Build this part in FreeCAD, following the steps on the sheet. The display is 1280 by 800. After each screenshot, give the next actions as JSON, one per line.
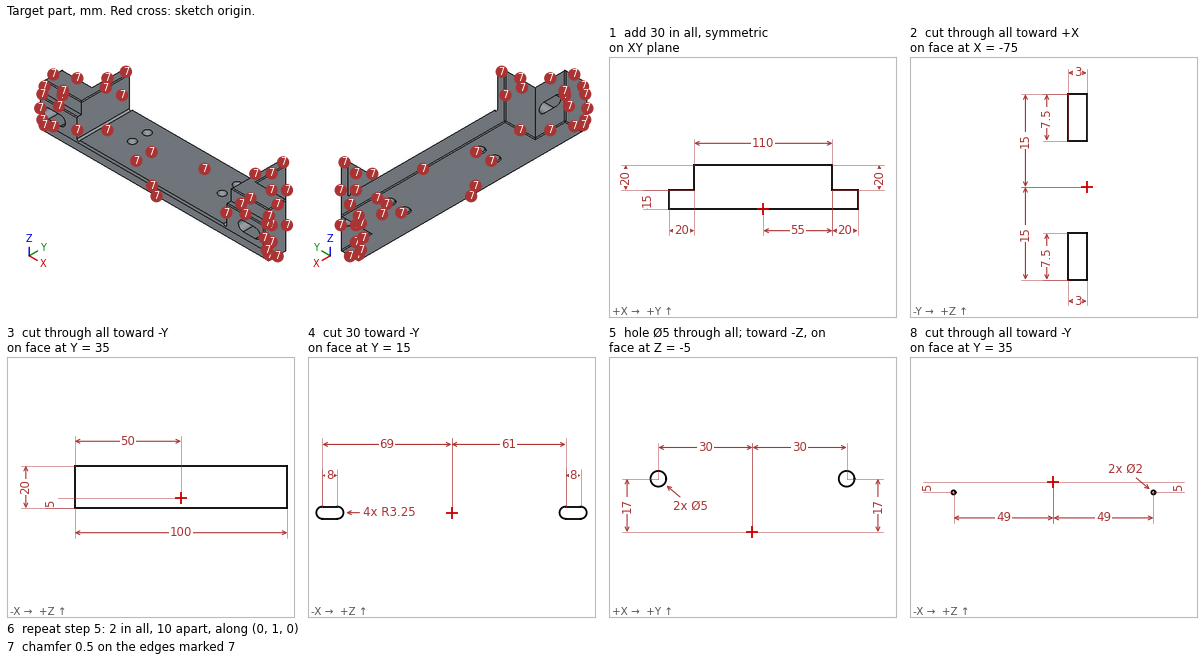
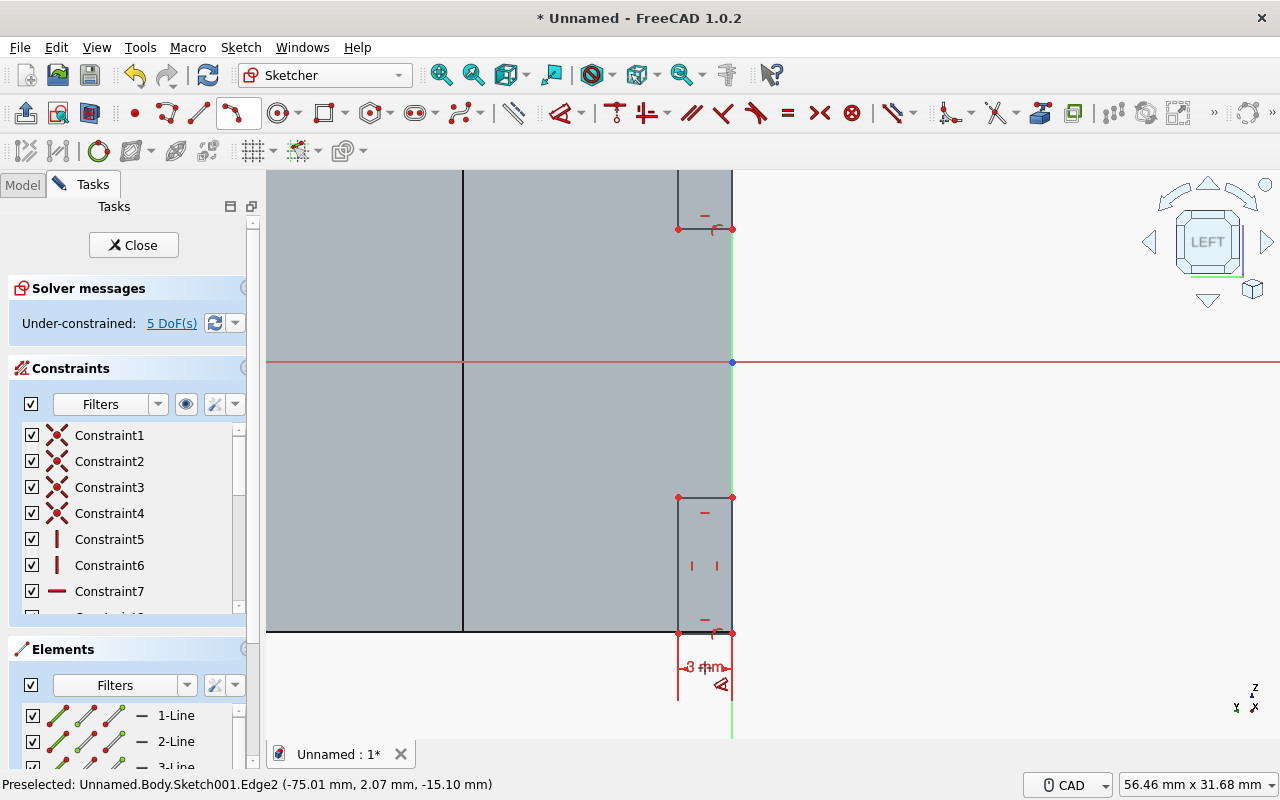
{"action": "left_click", "coordinate": [695, 229]}
{"action": "left_click", "coordinate": [705, 263]}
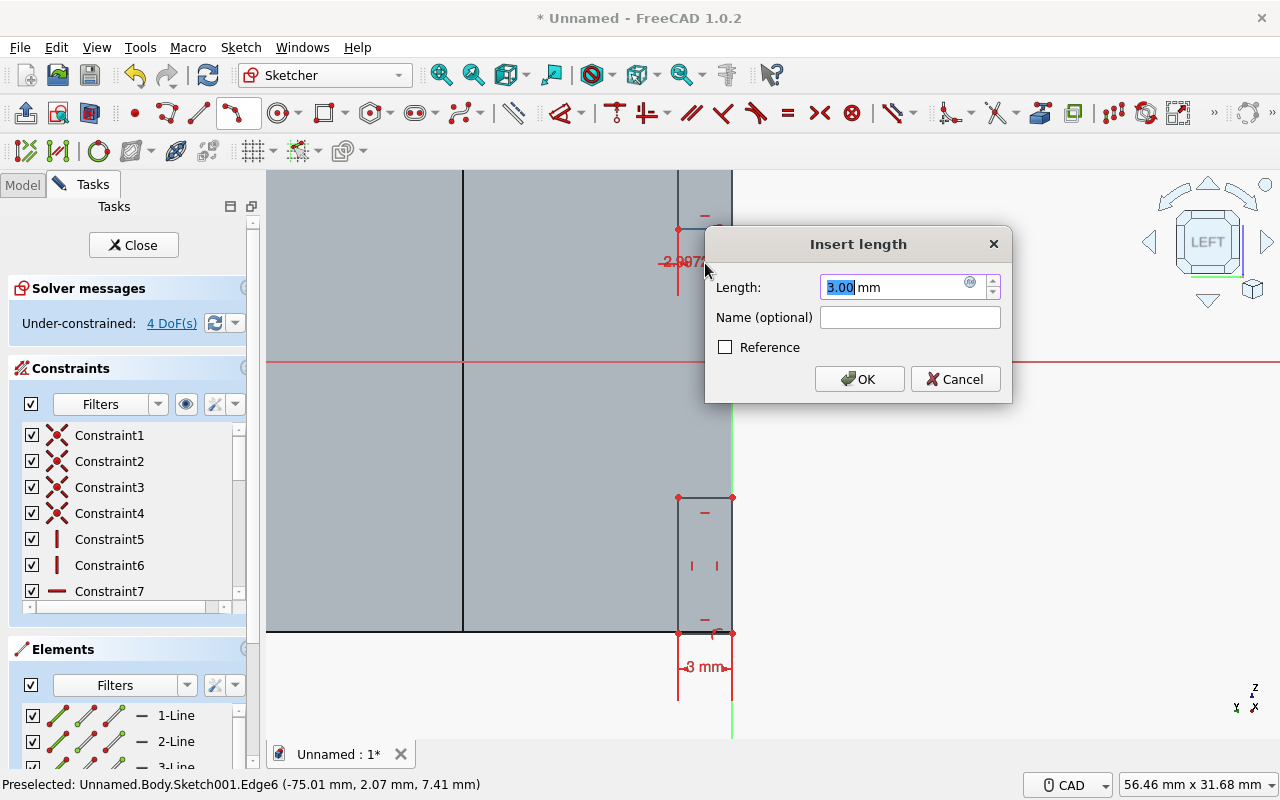
{"action": "type", "text": "3"}
{"action": "key", "text": "Return"}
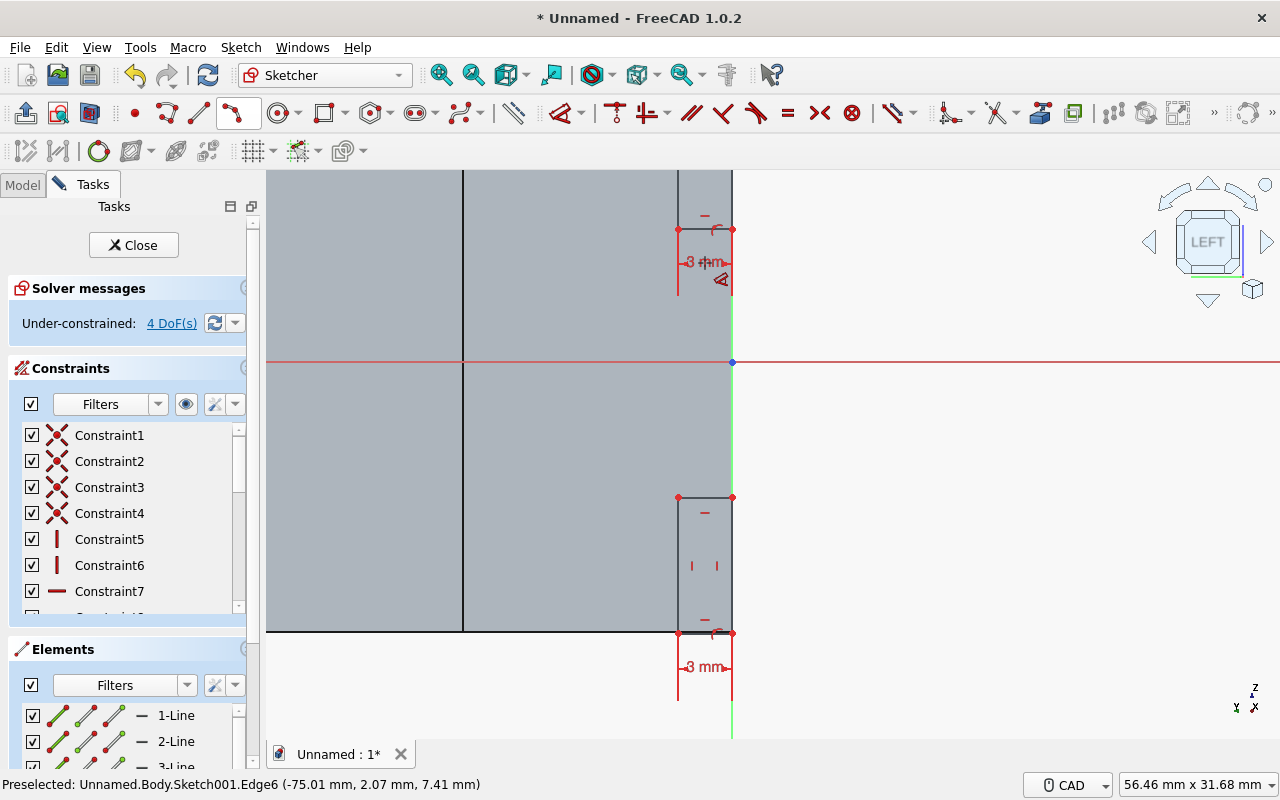
{"action": "left_click", "coordinate": [678, 539]}
{"action": "left_click", "coordinate": [644, 566]}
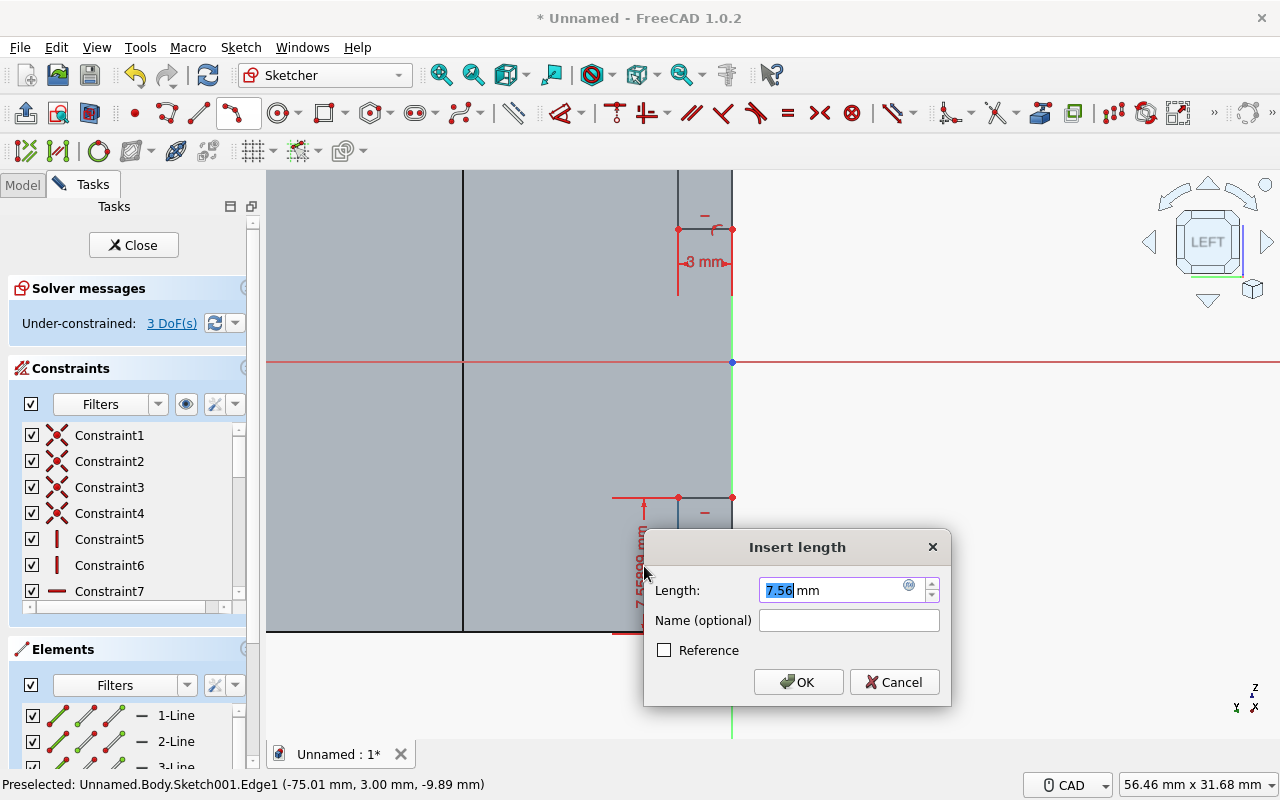
{"action": "type", "text": "7.5"}
{"action": "key", "text": "Return"}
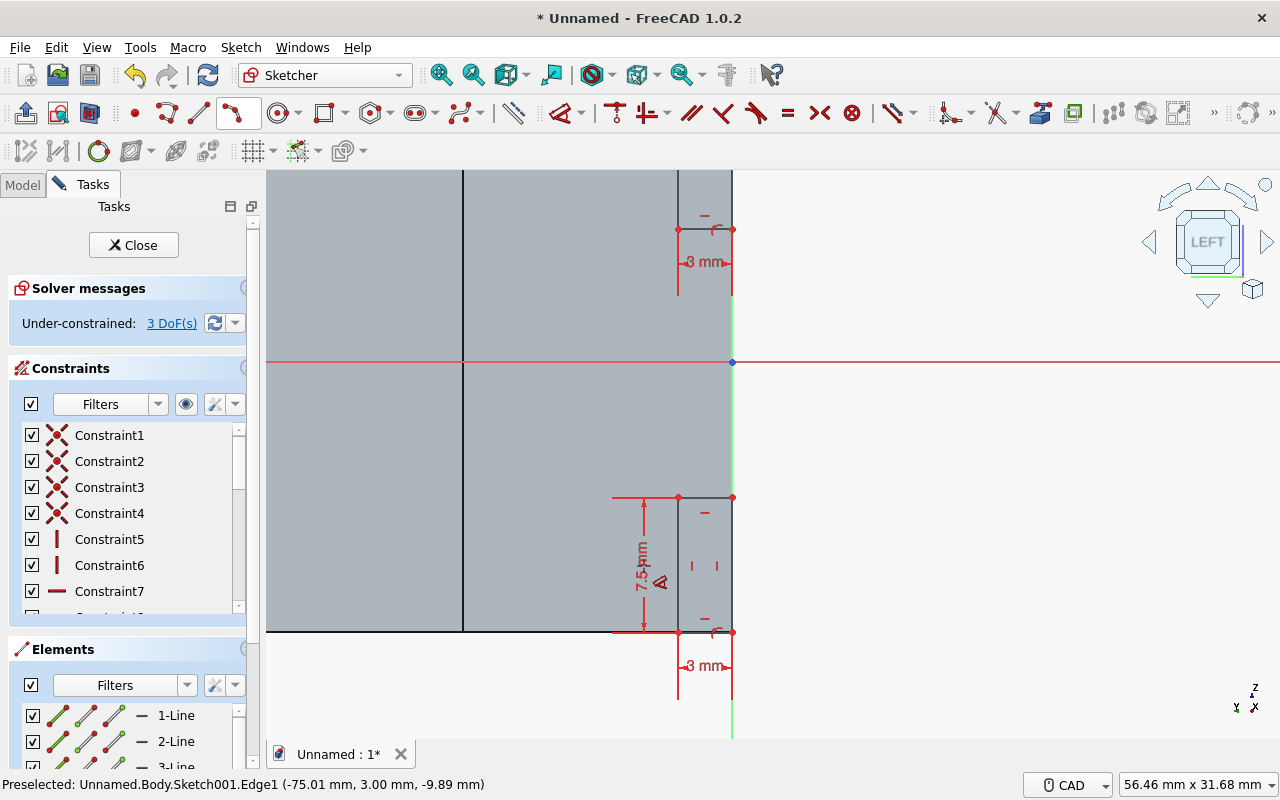
{"action": "left_click", "coordinate": [678, 202]}
{"action": "left_click", "coordinate": [644, 214]}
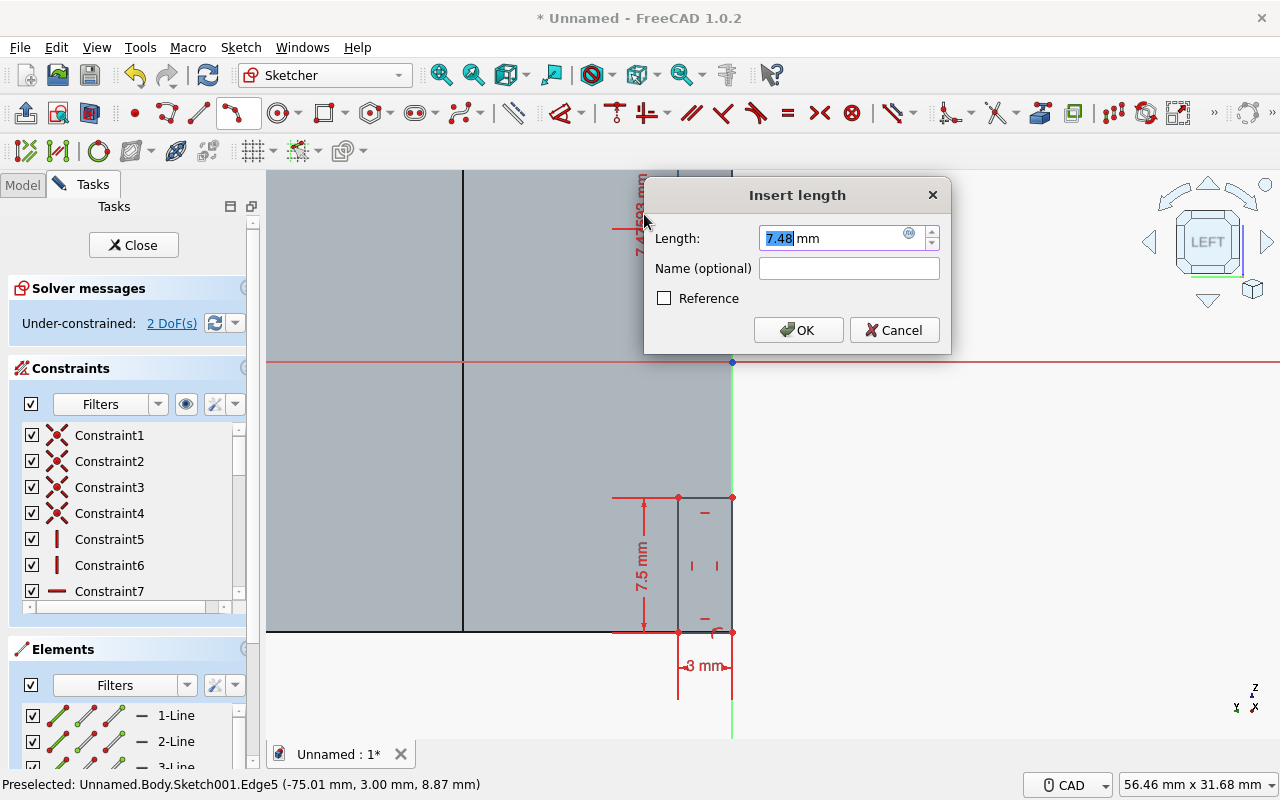
{"action": "type", "text": "7.5"}
{"action": "key", "text": "Return"}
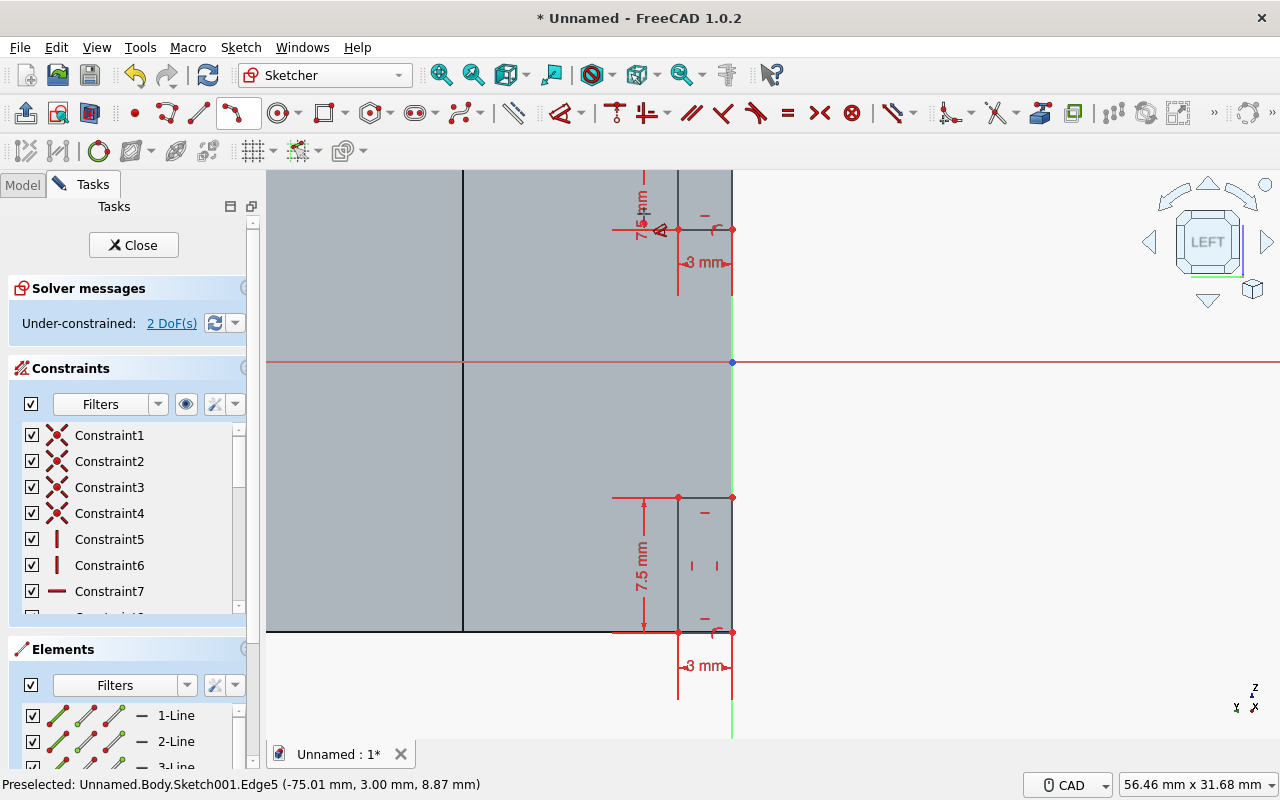
{"action": "left_click", "coordinate": [678, 633]}
{"action": "left_click", "coordinate": [766, 497]}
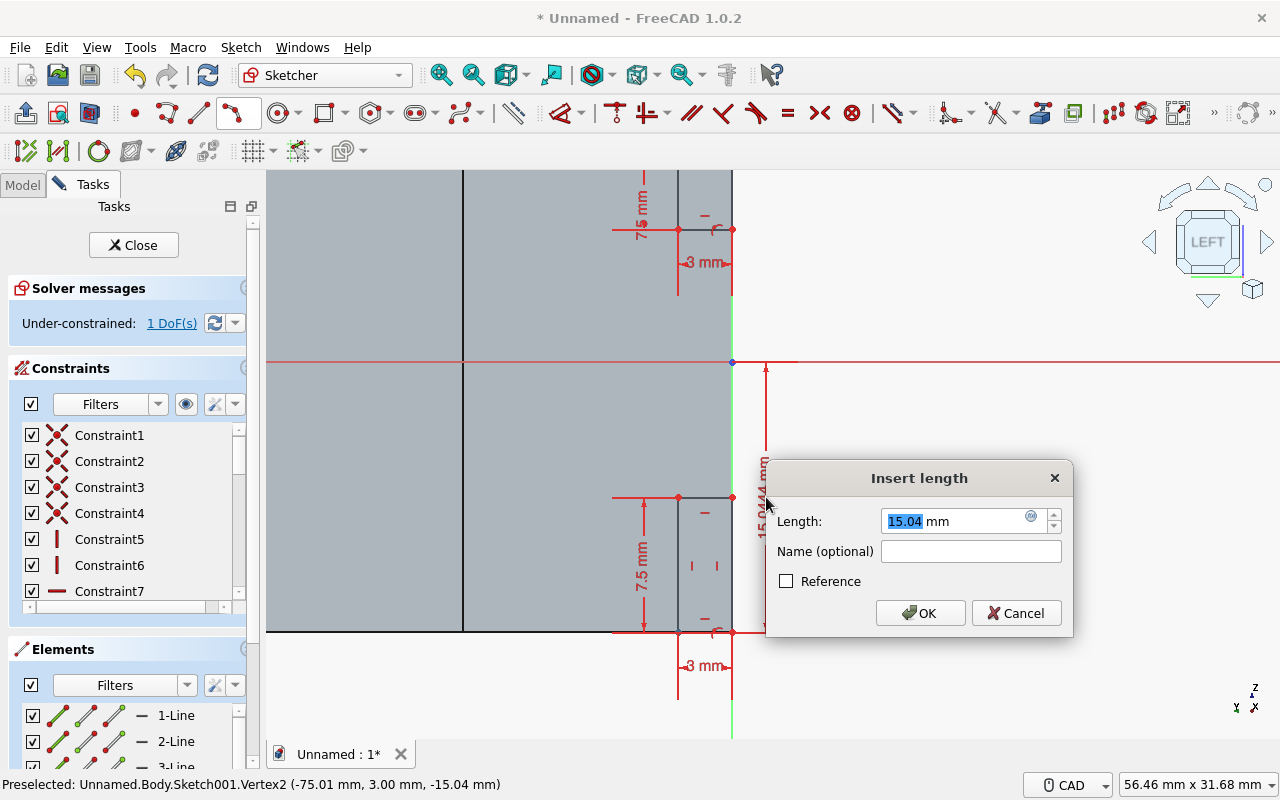
{"action": "type", "text": "15"}
{"action": "key", "text": "Return"}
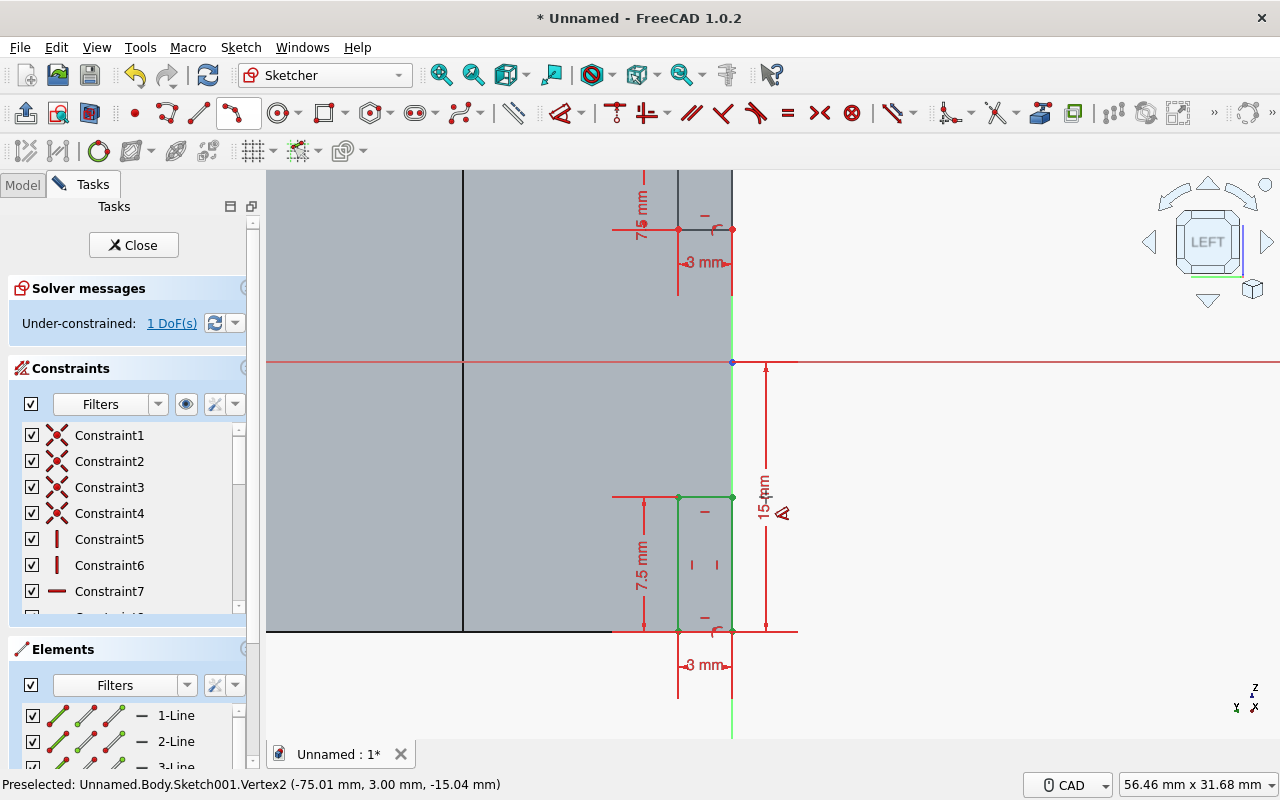
{"action": "scroll", "coordinate": [703, 642], "scroll_direction": "down", "scroll_amount": 2}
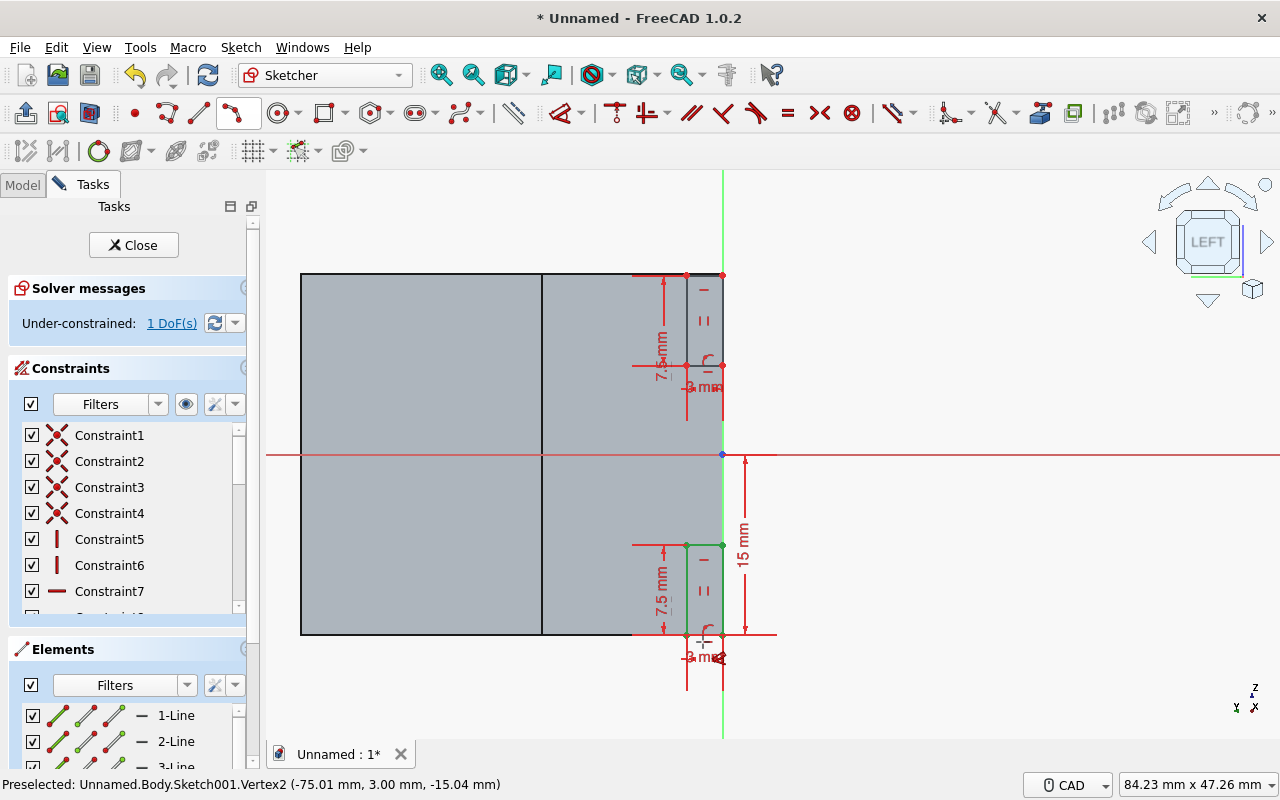
{"action": "left_click", "coordinate": [687, 276]}
{"action": "left_click", "coordinate": [757, 365]}